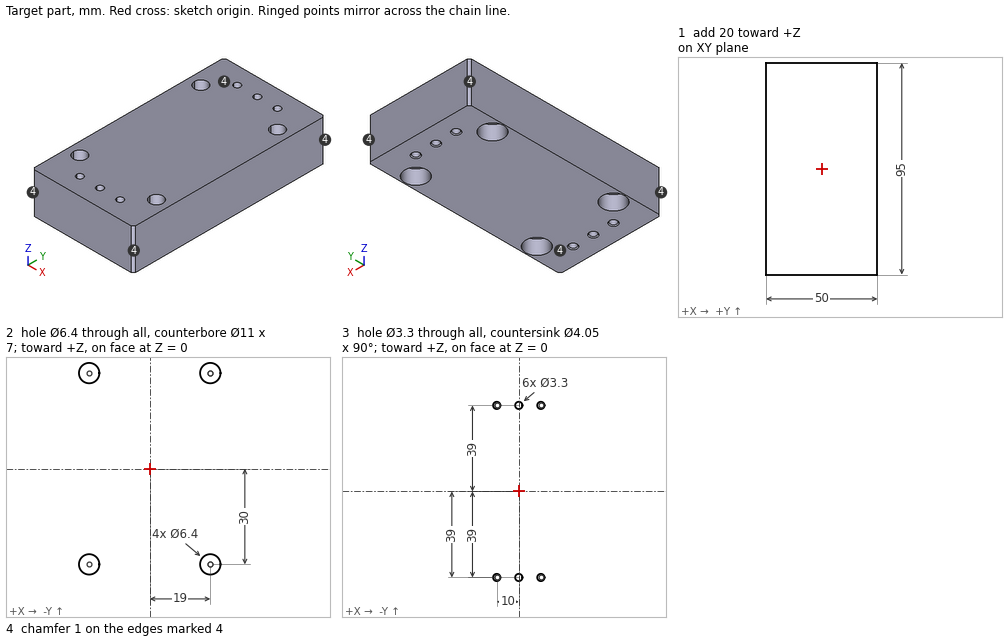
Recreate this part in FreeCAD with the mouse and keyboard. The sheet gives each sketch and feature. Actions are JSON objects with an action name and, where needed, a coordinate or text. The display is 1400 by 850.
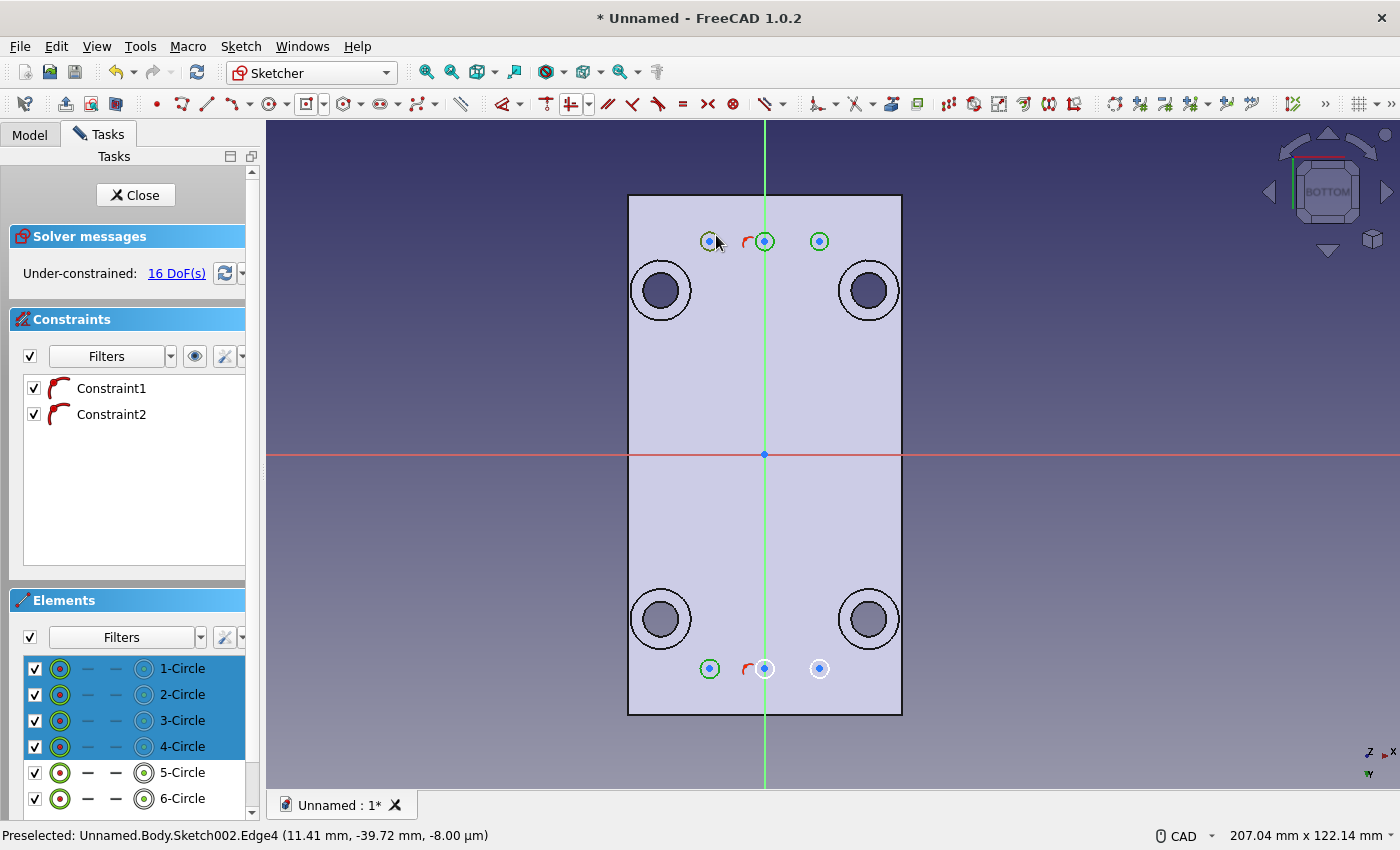
{"action": "scroll", "coordinate": [826, 662], "scroll_direction": "up", "scroll_amount": 3}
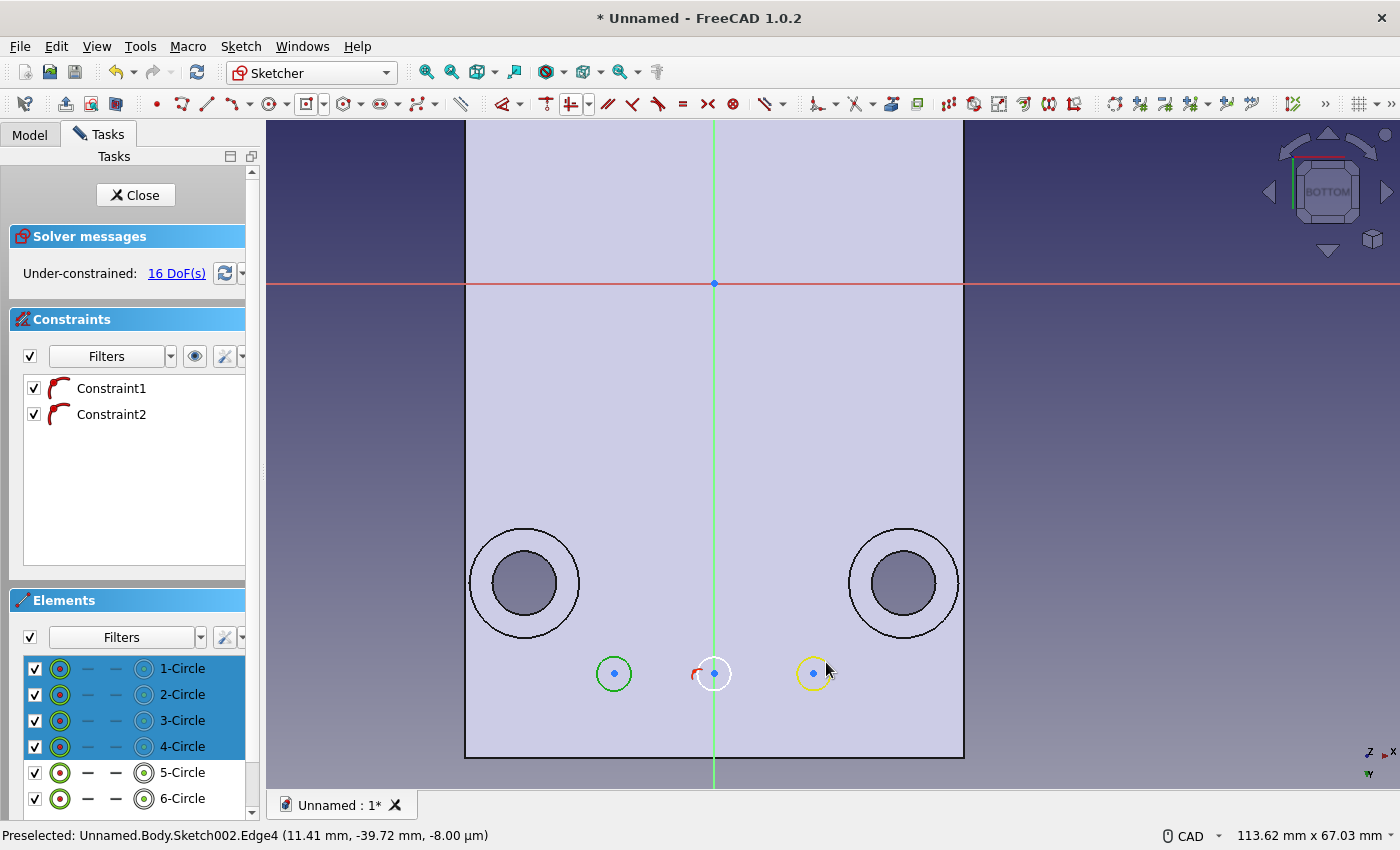
{"action": "left_click", "coordinate": [826, 662]}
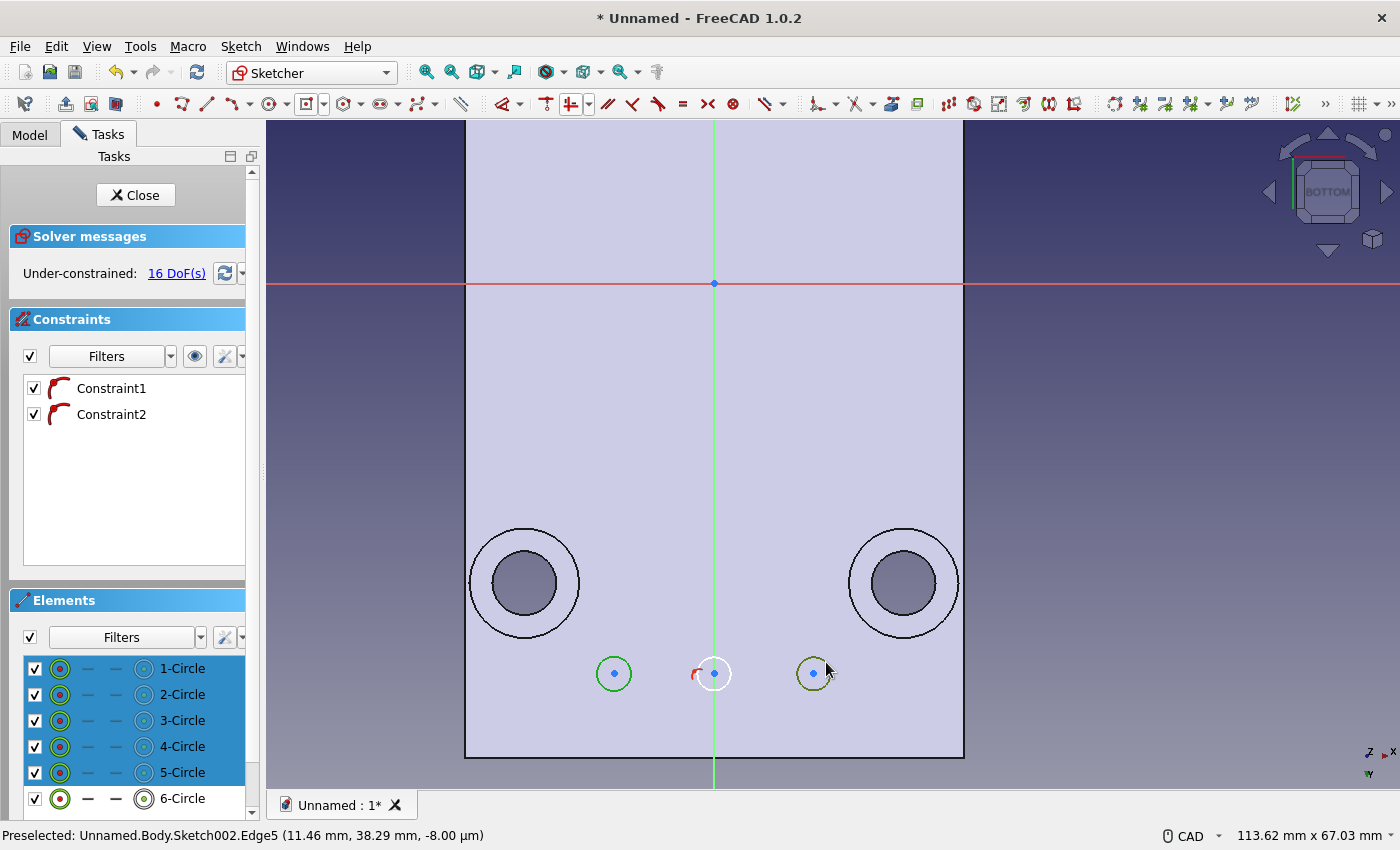
{"action": "left_click", "coordinate": [726, 662]}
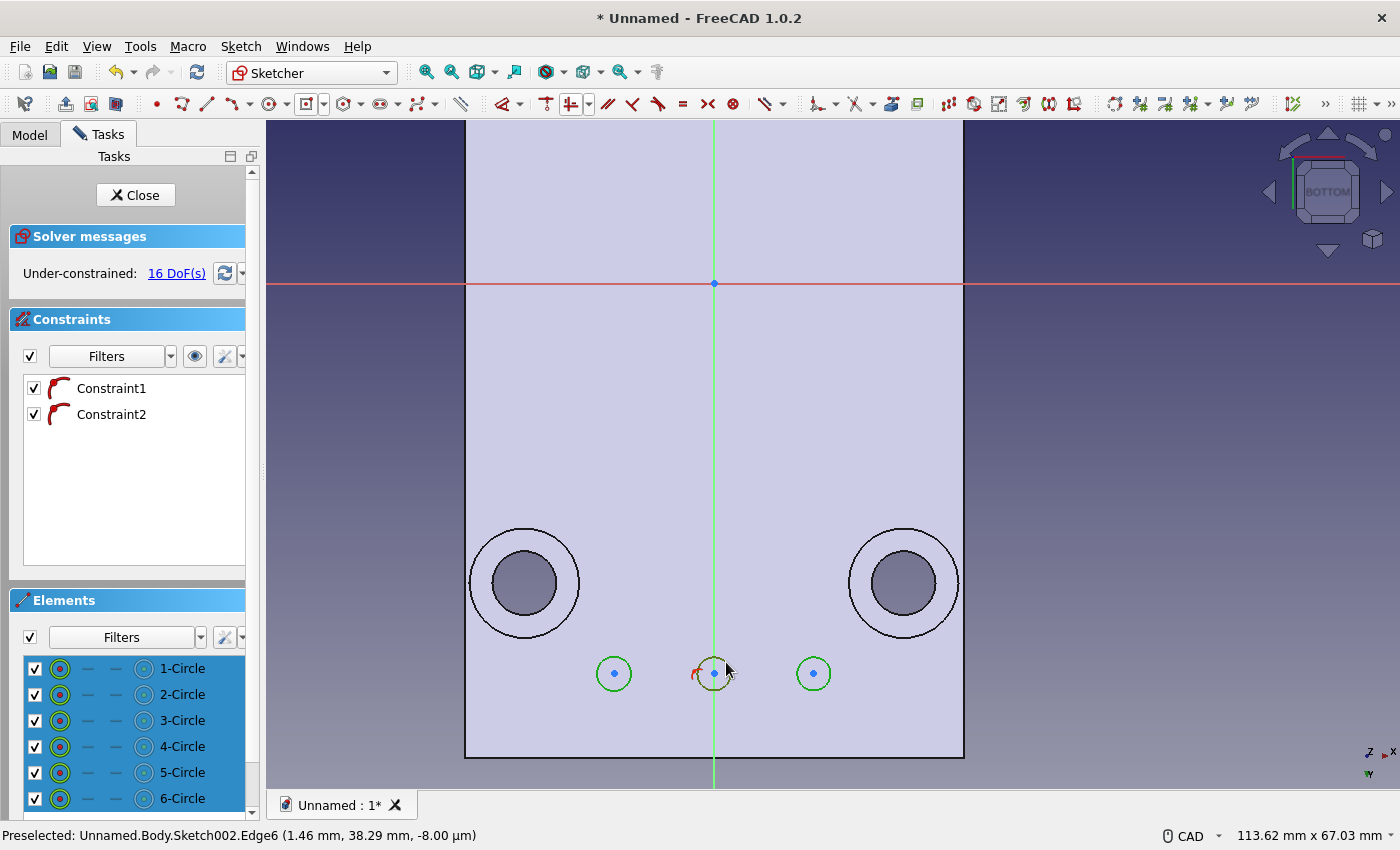
{"action": "left_click", "coordinate": [683, 104]}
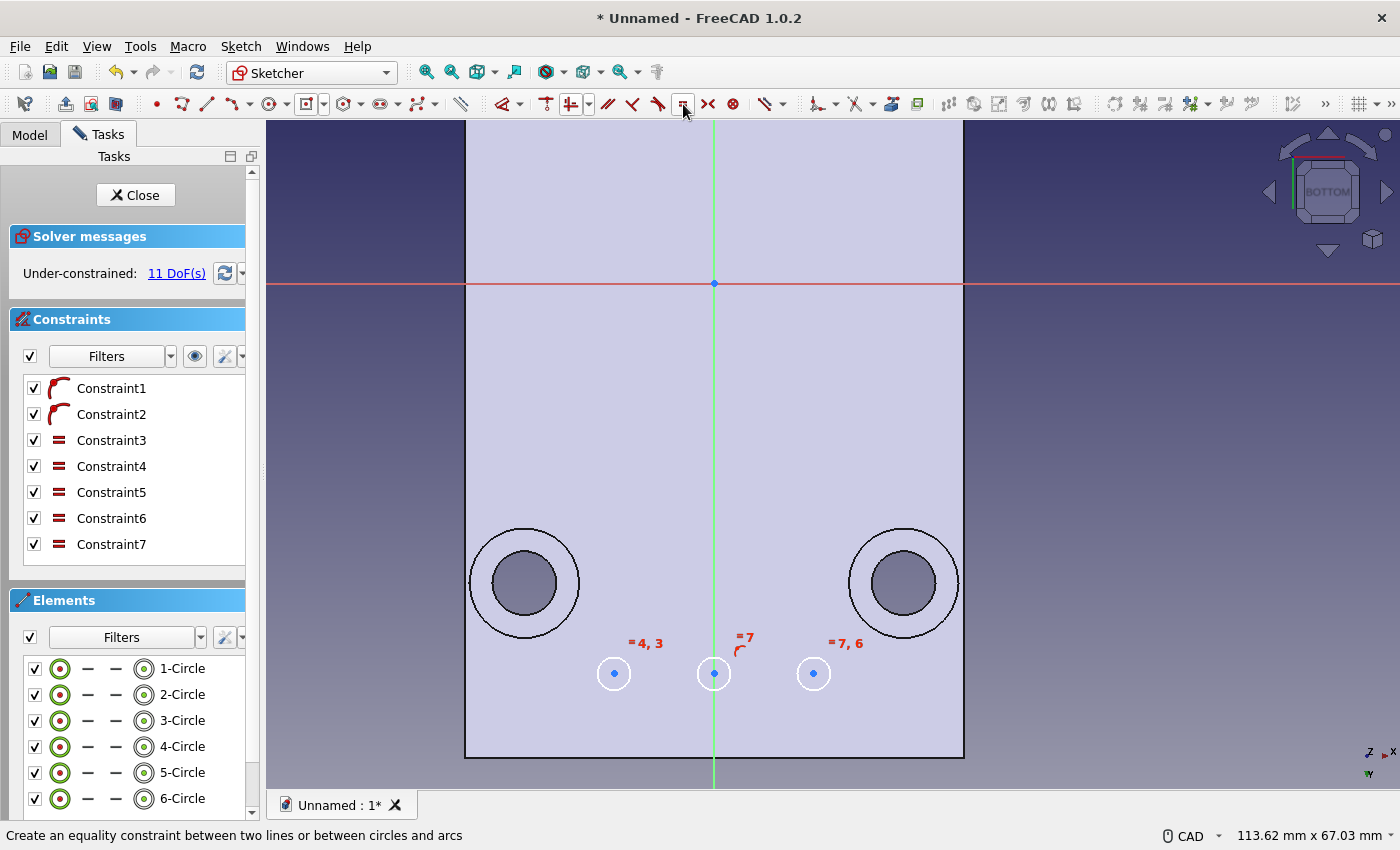
{"action": "left_click", "coordinate": [614, 674]}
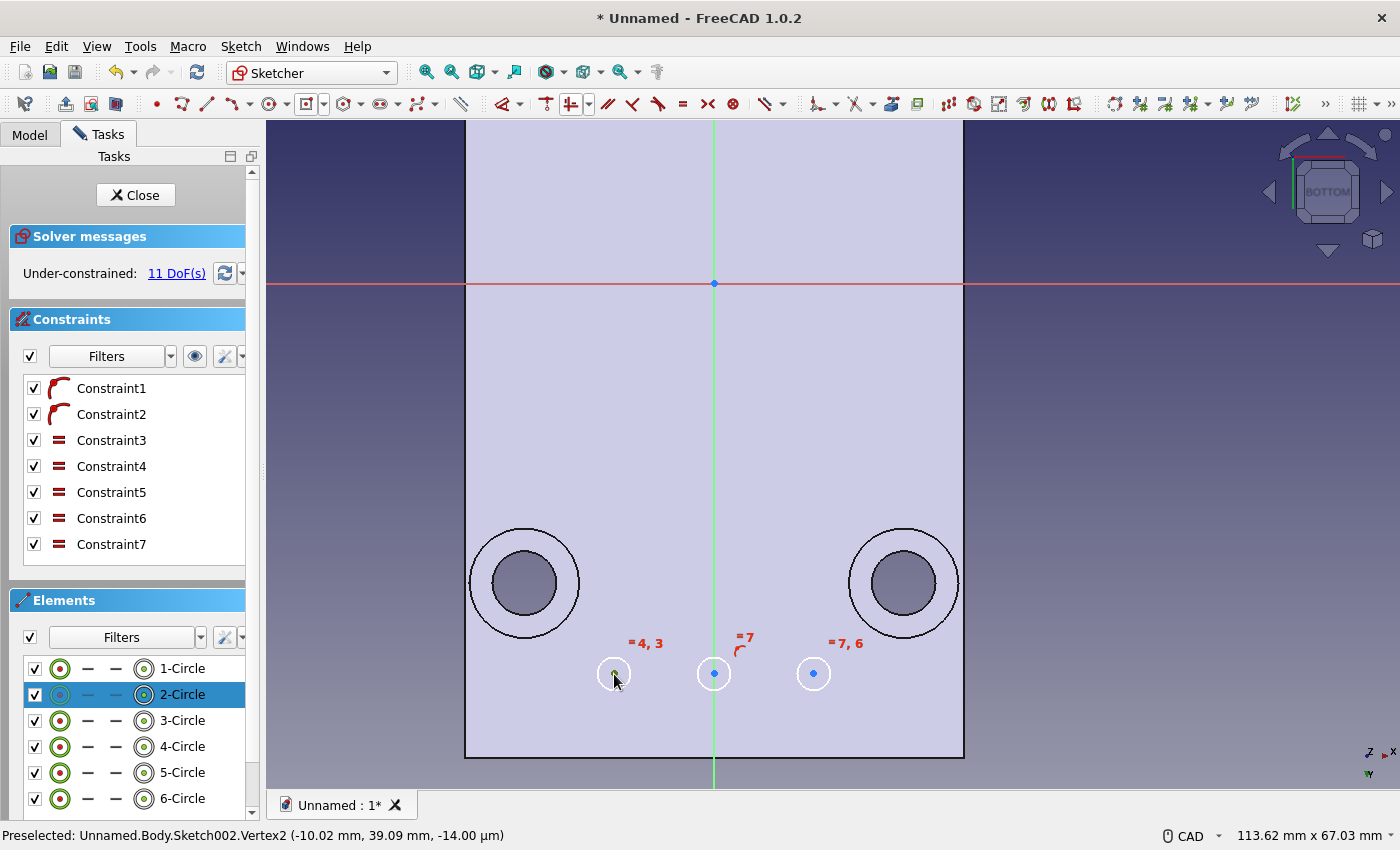
{"action": "scroll", "coordinate": [826, 662], "scroll_direction": "down", "scroll_amount": 3}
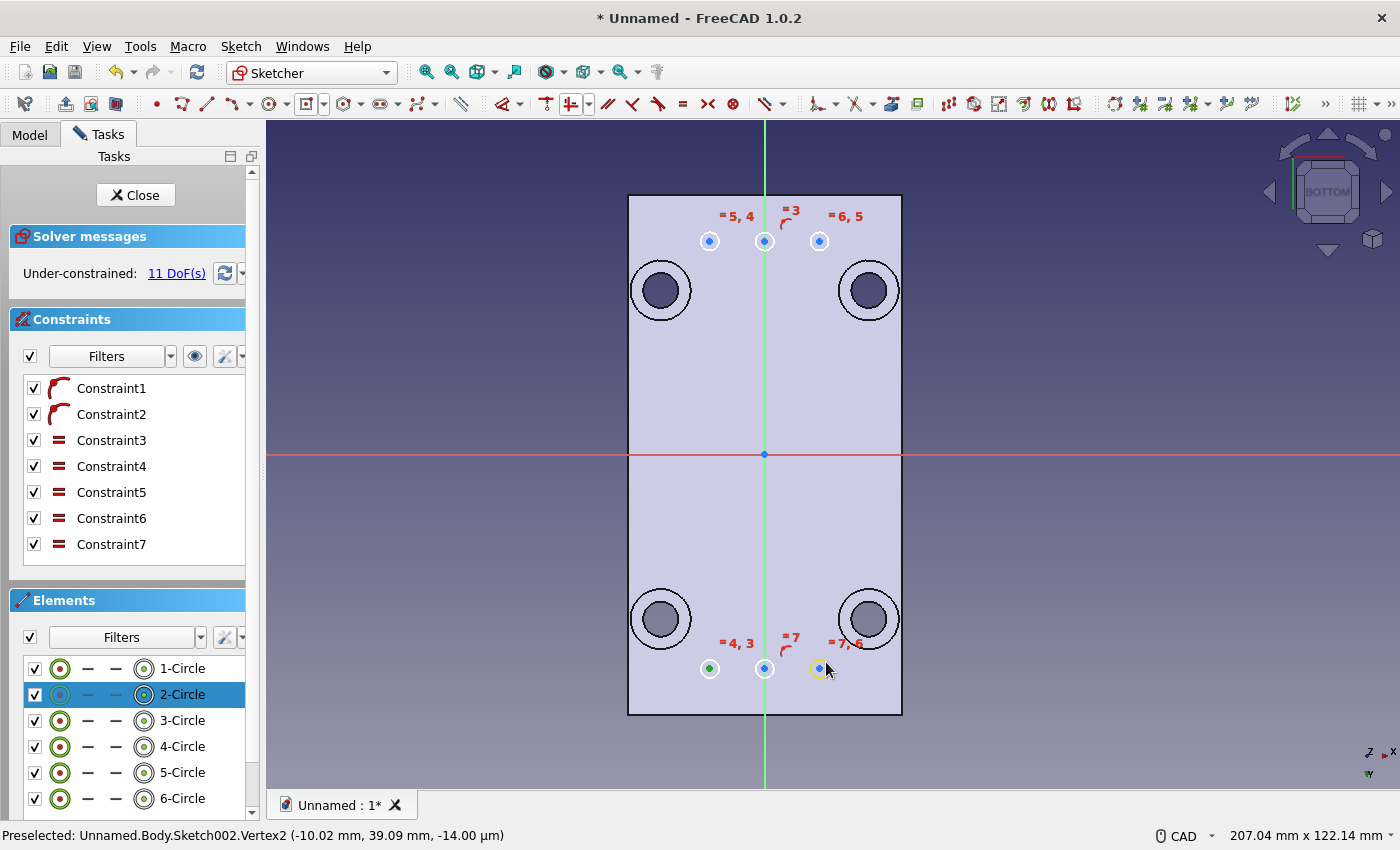
{"action": "left_click", "coordinate": [710, 241]}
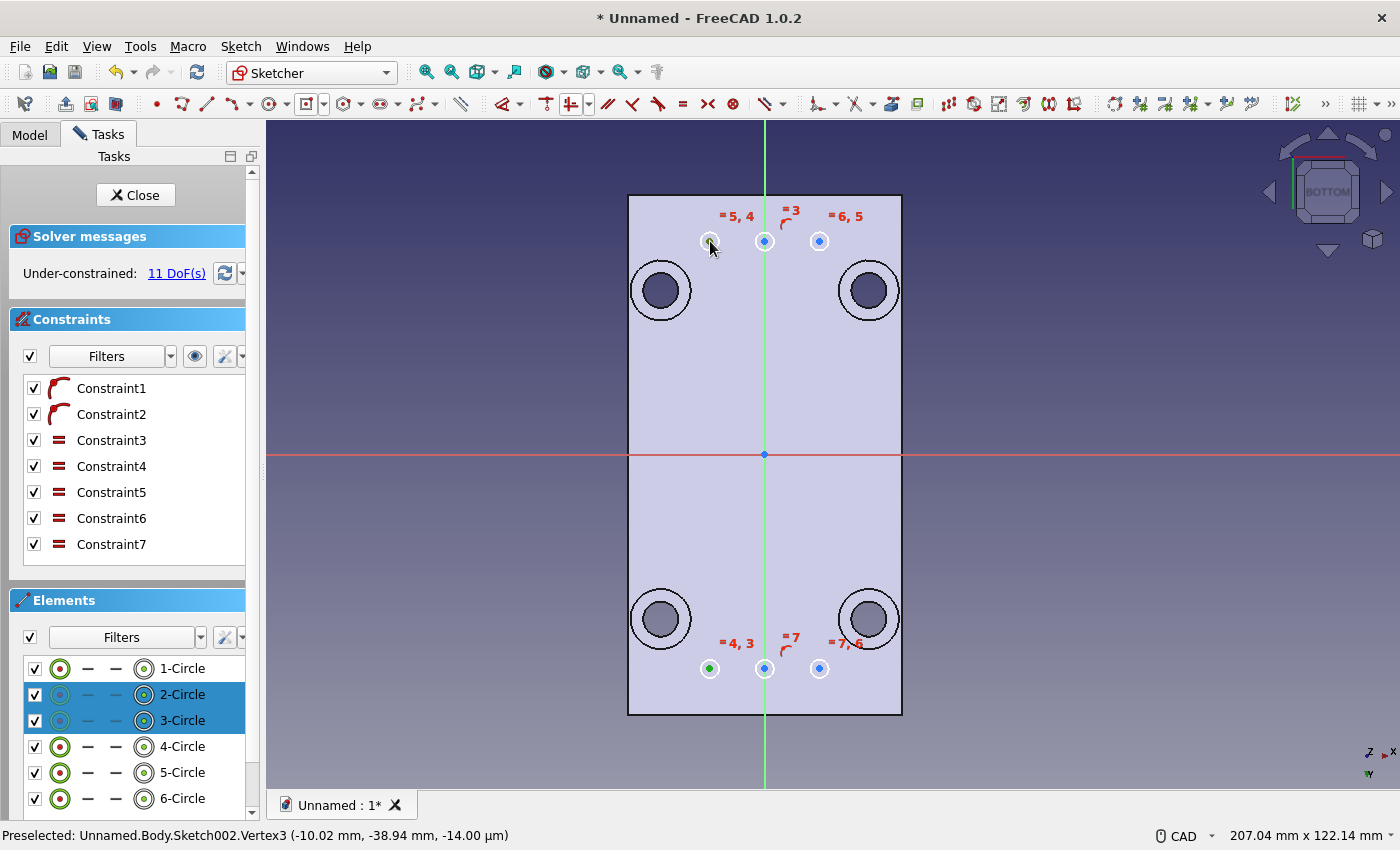
{"action": "left_click", "coordinate": [361, 455]}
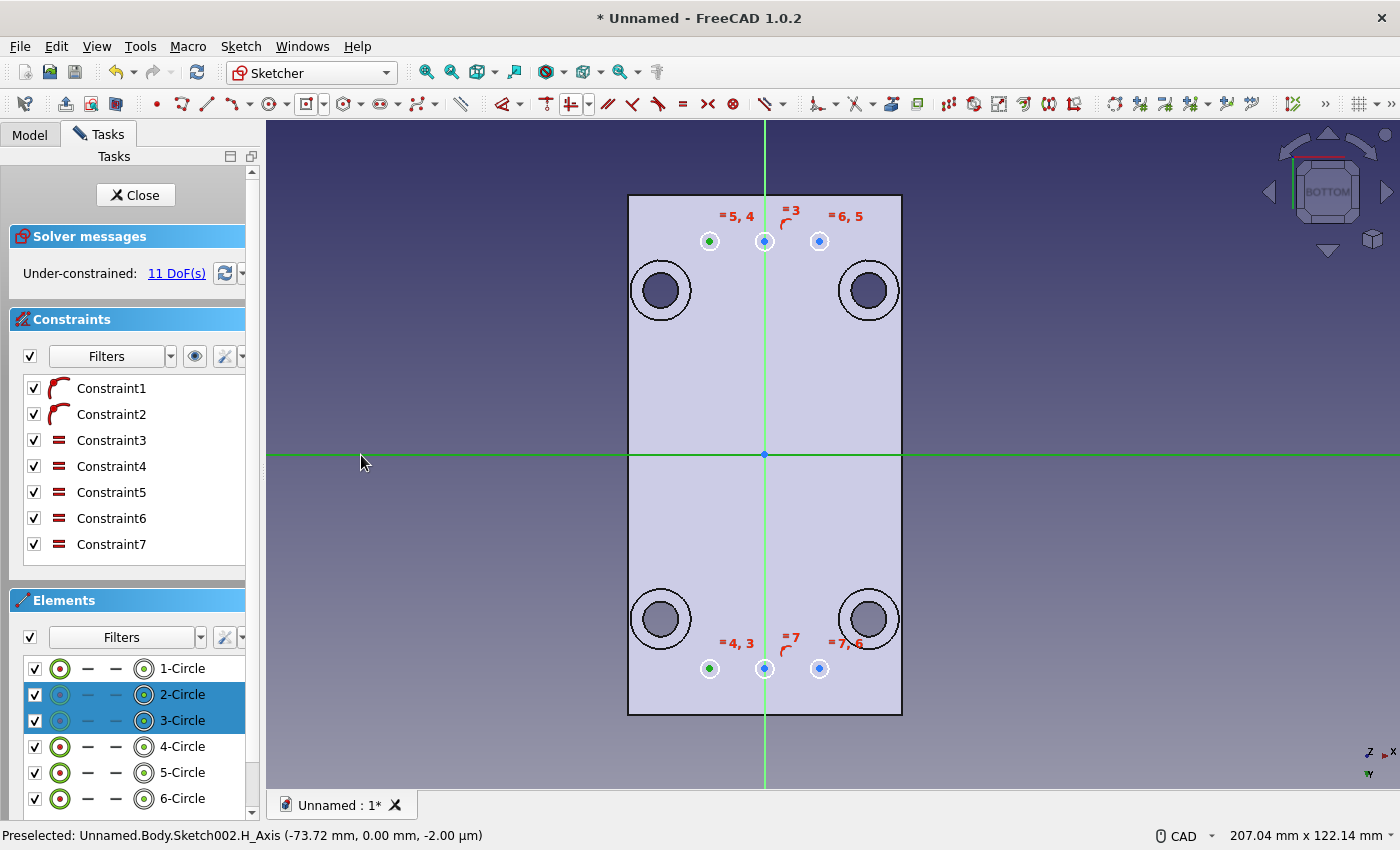
{"action": "left_click", "coordinate": [708, 104]}